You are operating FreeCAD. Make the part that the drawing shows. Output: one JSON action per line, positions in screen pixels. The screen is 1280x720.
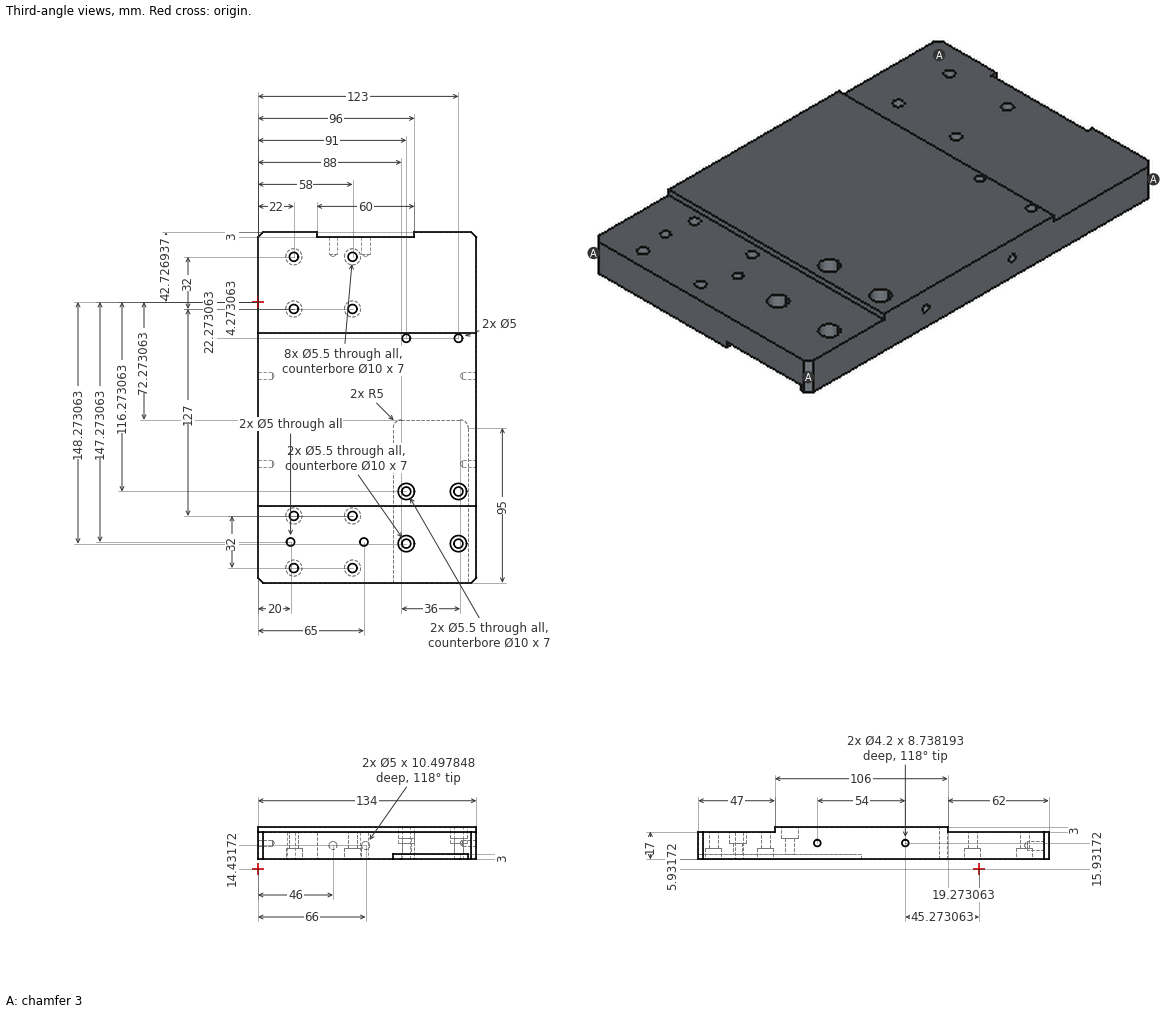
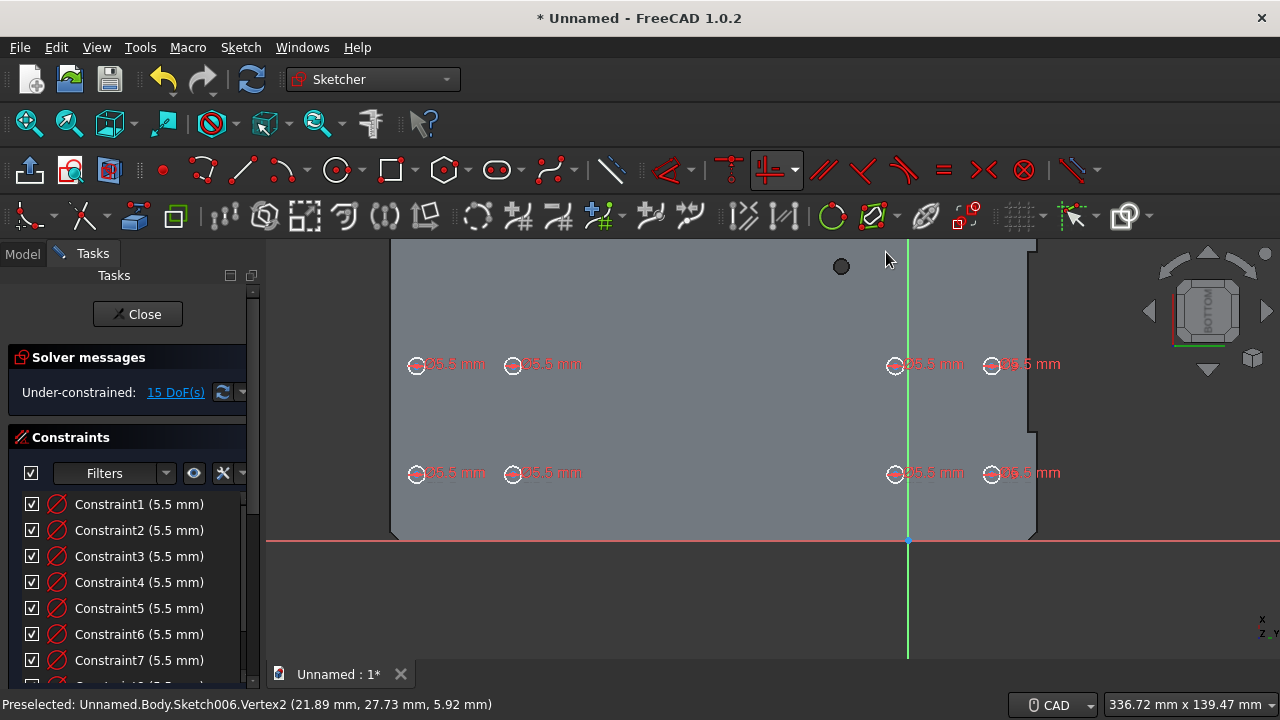
{"action": "left_click", "coordinate": [992, 475]}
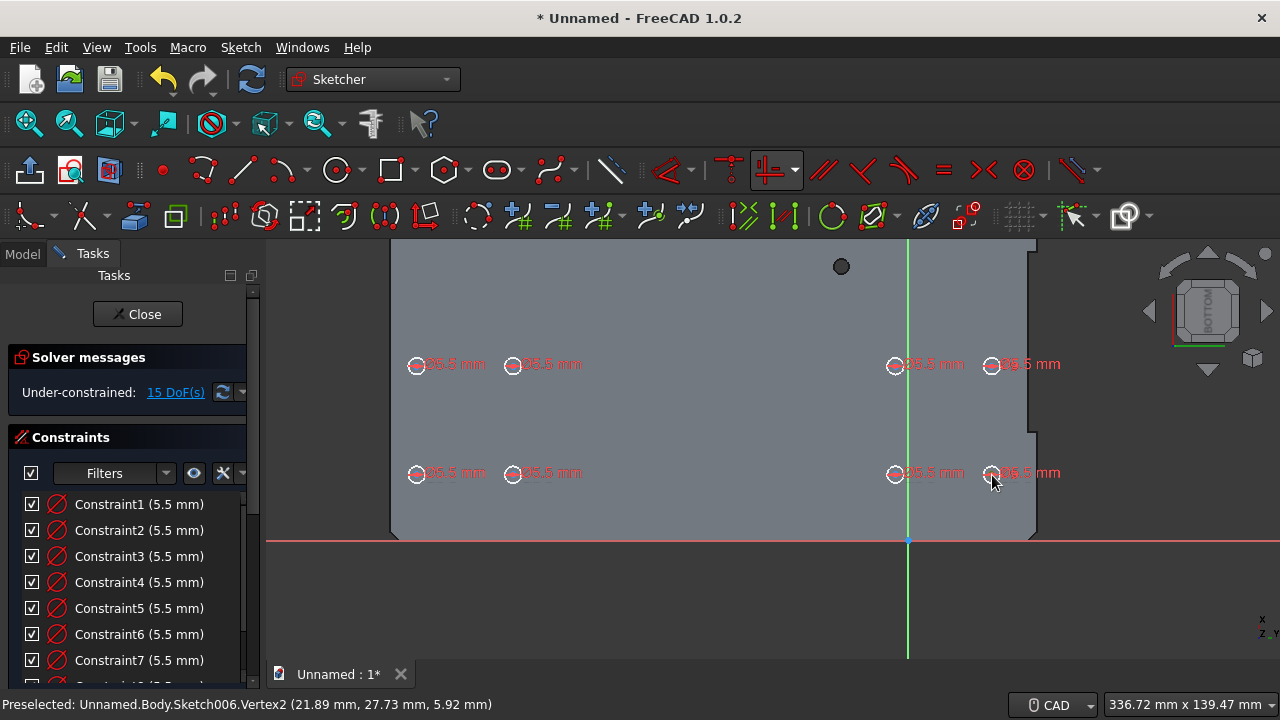
{"action": "left_click", "coordinate": [896, 475]}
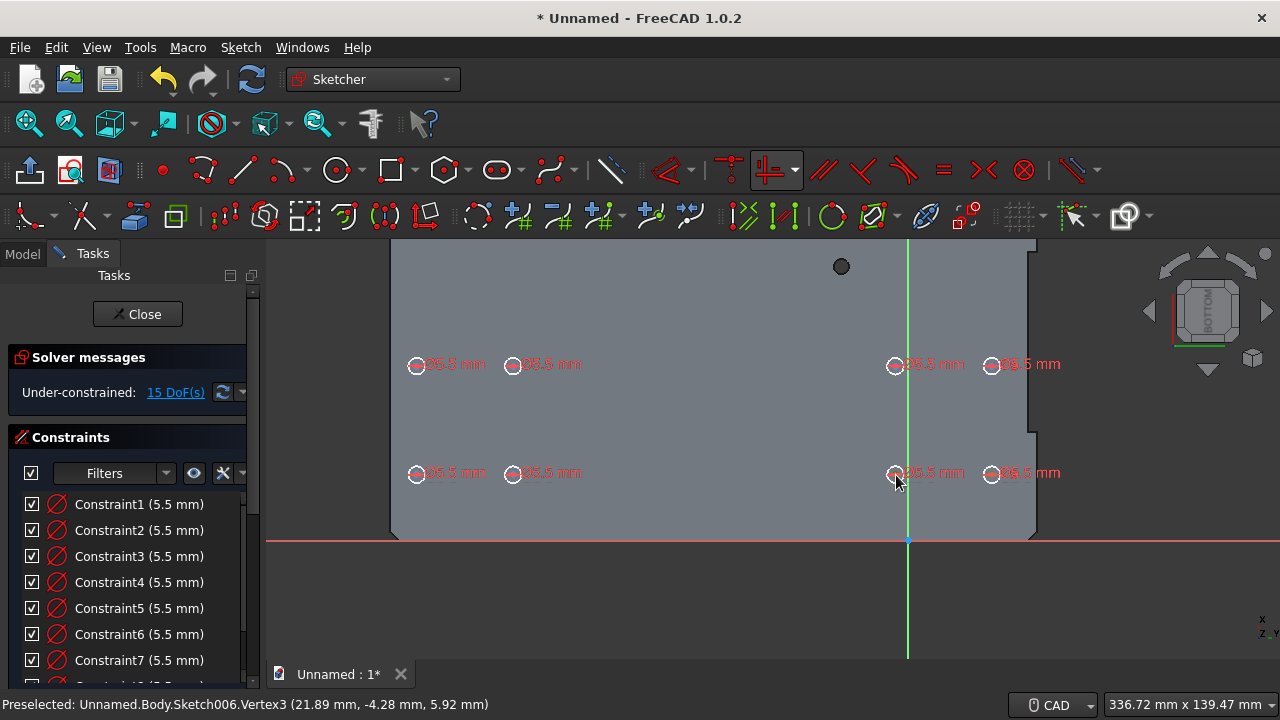
{"action": "left_click", "coordinate": [798, 170]}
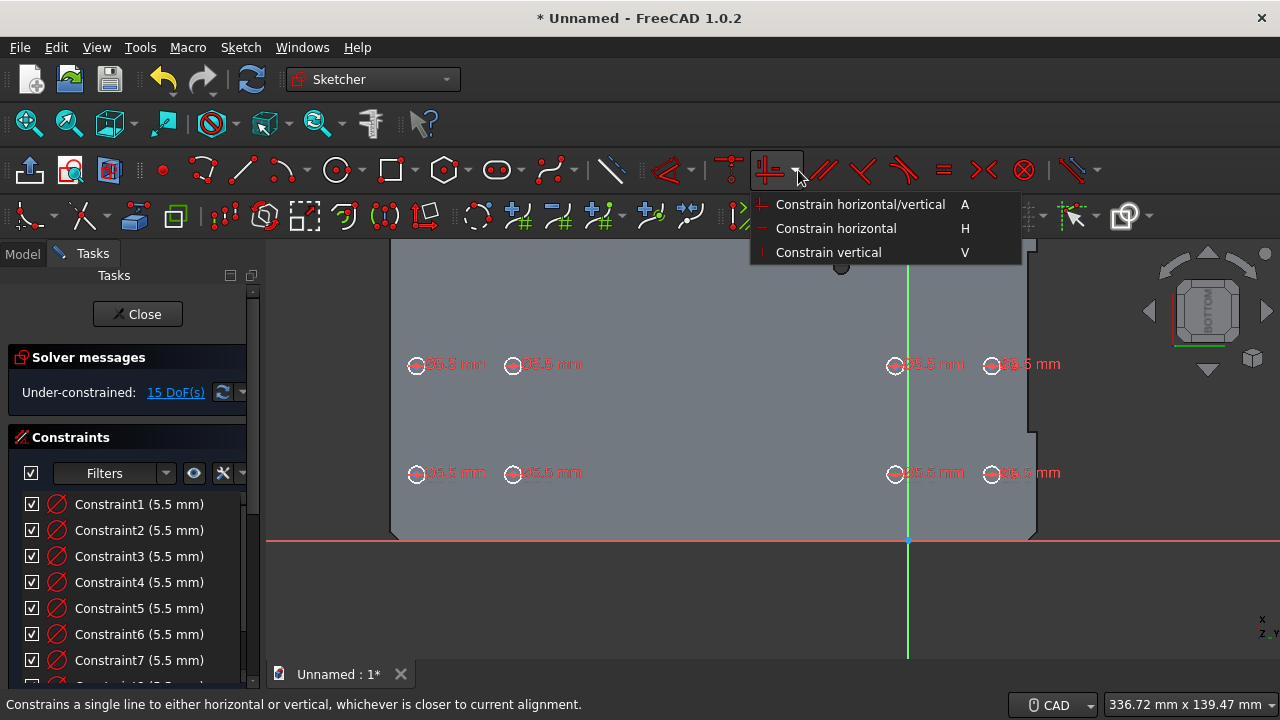
{"action": "left_click", "coordinate": [886, 228]}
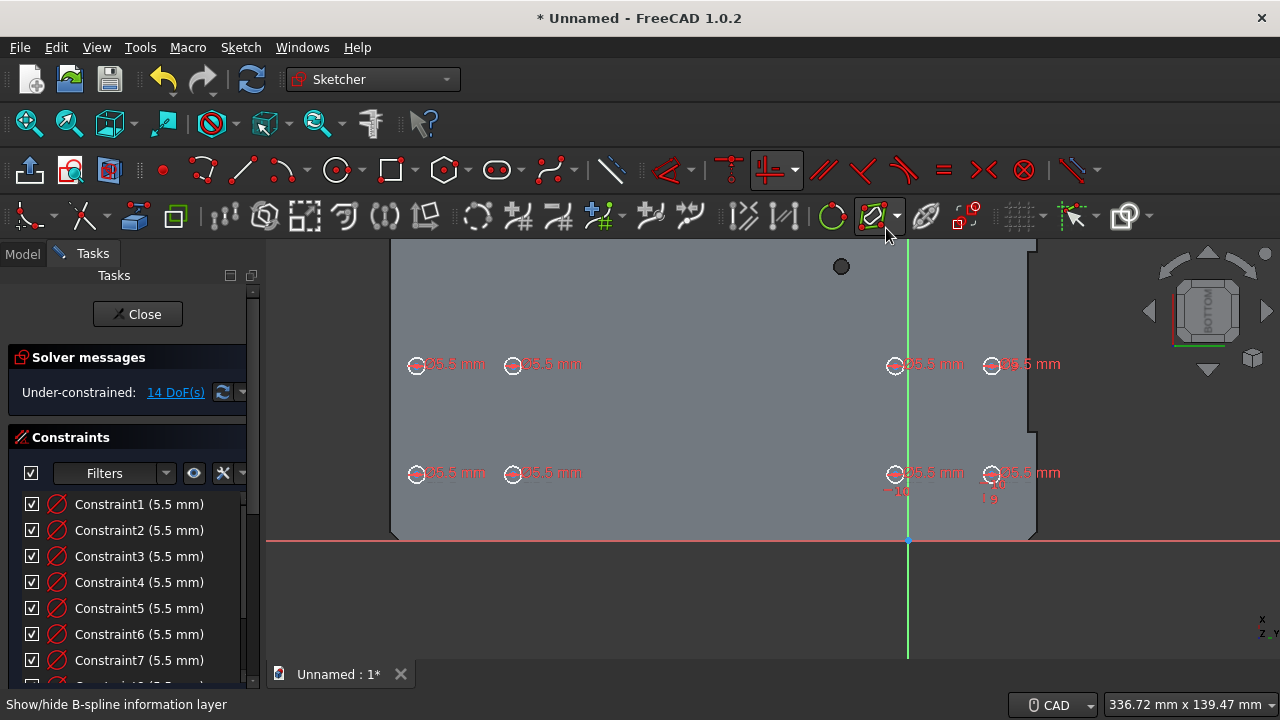
{"action": "left_click", "coordinate": [896, 475]}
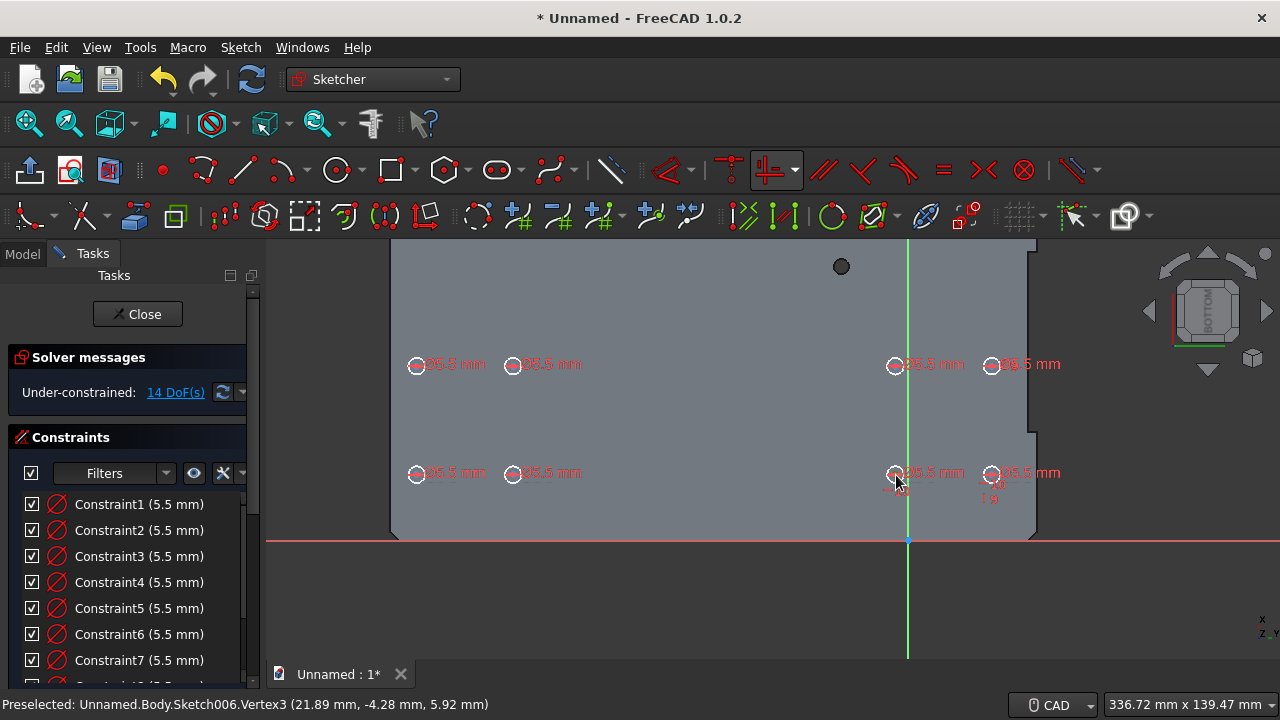
{"action": "left_click", "coordinate": [895, 366]}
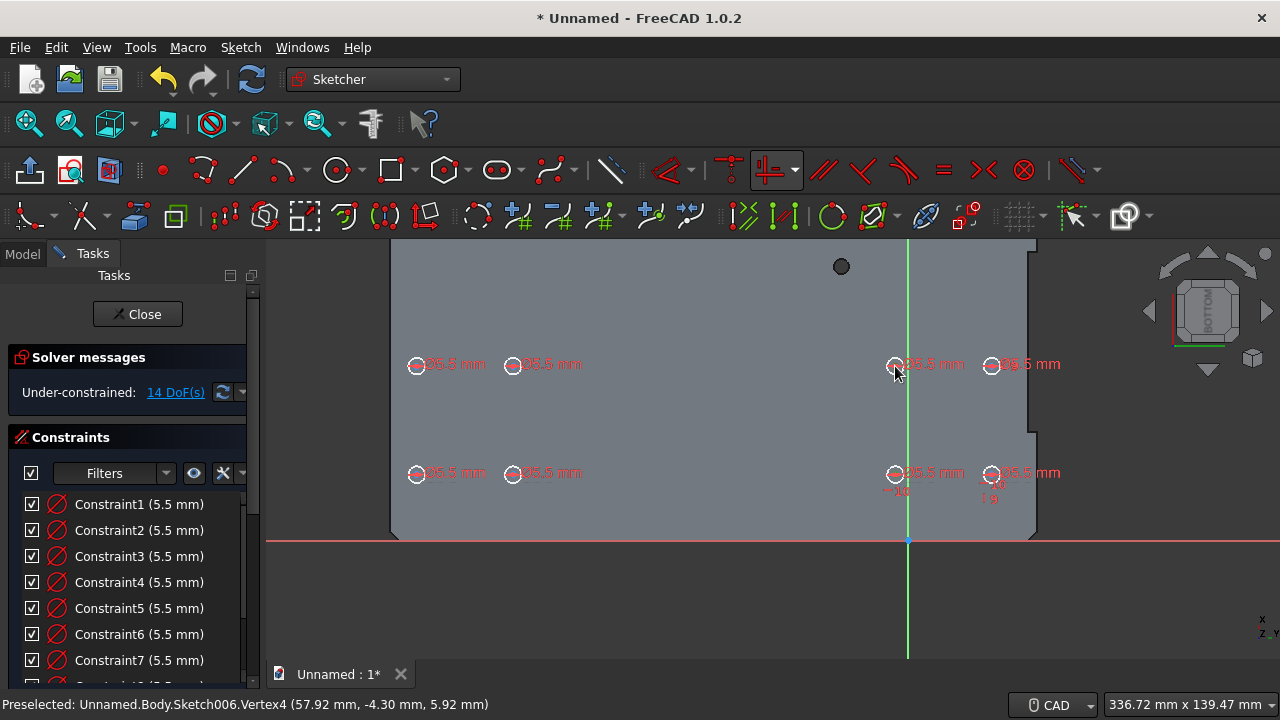
{"action": "left_click", "coordinate": [798, 170]}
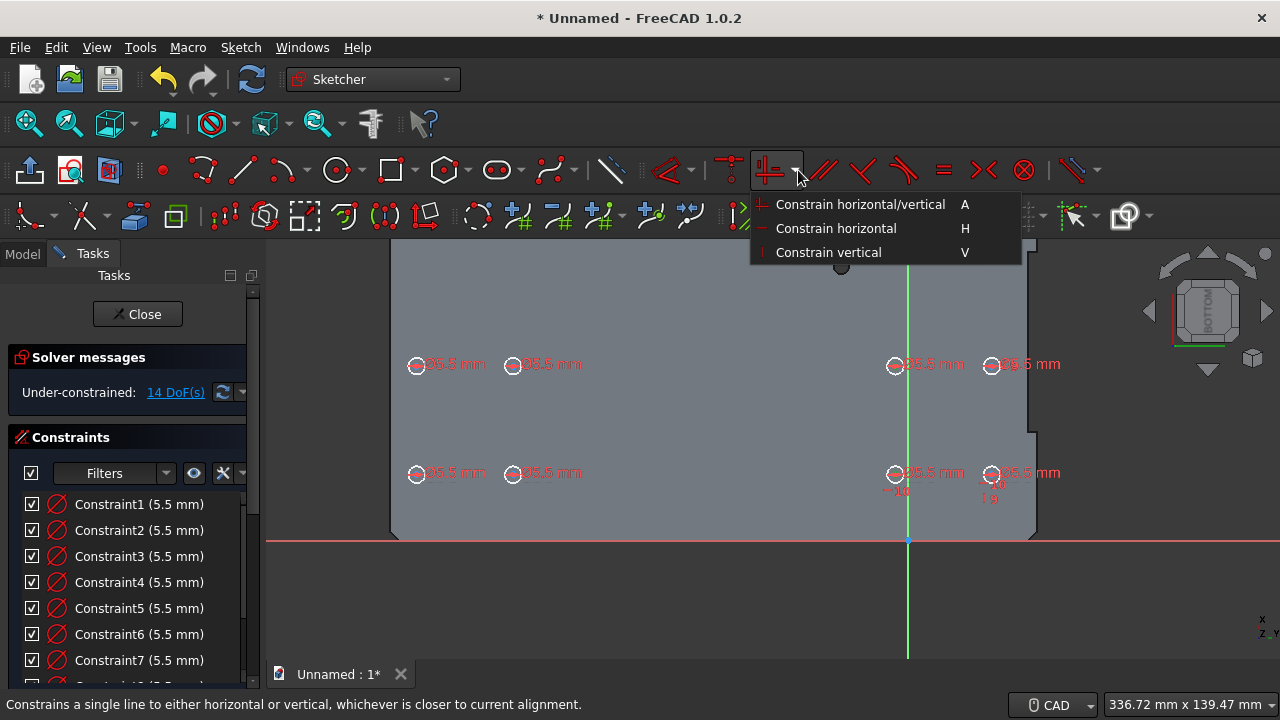
{"action": "left_click", "coordinate": [886, 252]}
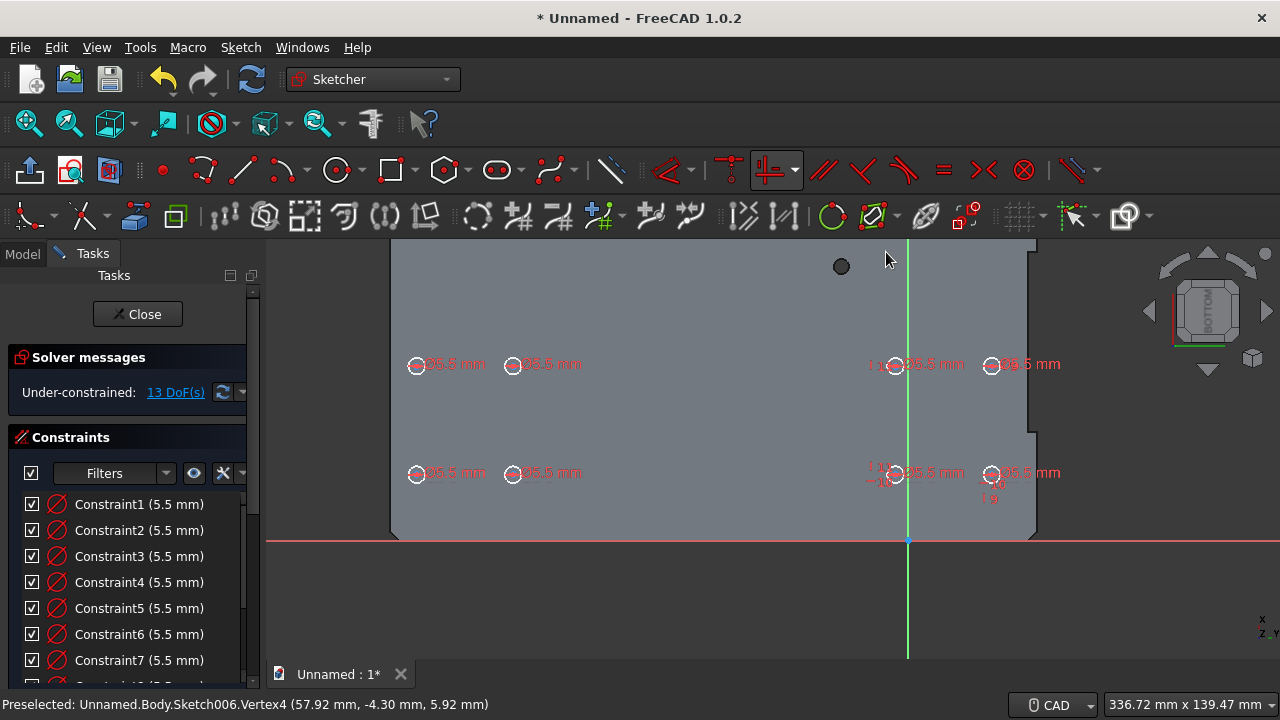
{"action": "left_click", "coordinate": [992, 366]}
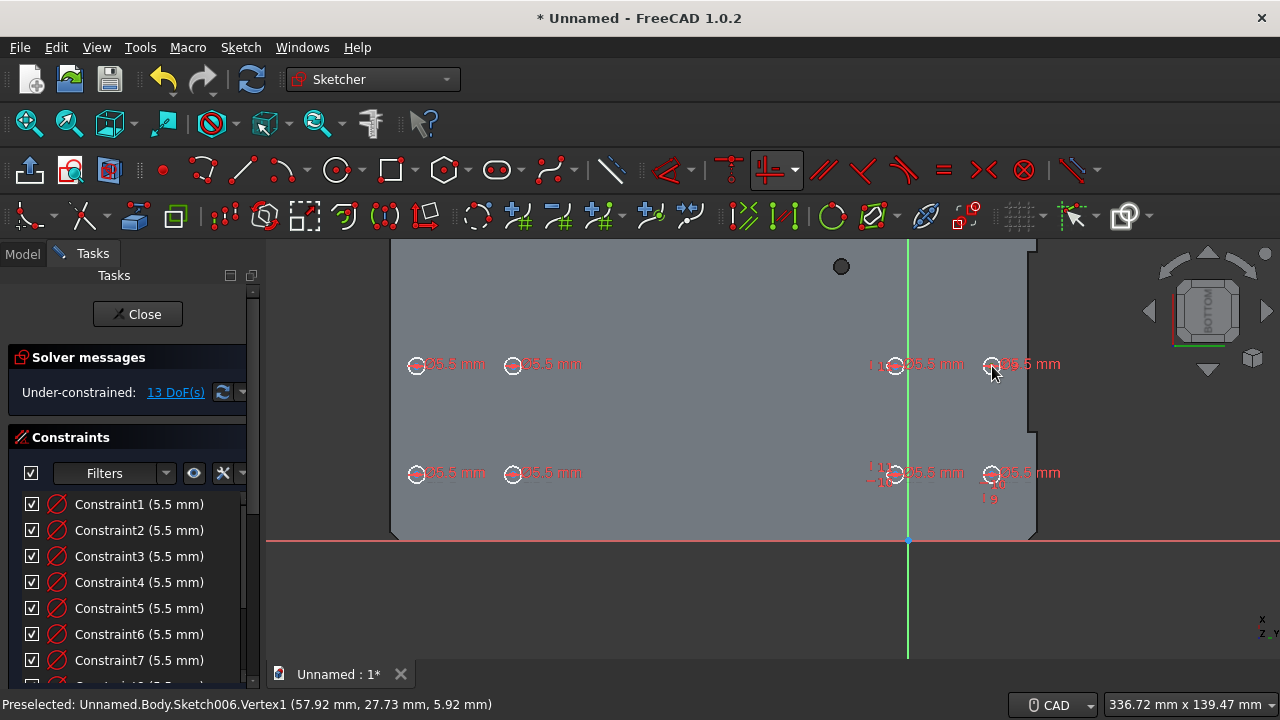
{"action": "left_click", "coordinate": [896, 366]}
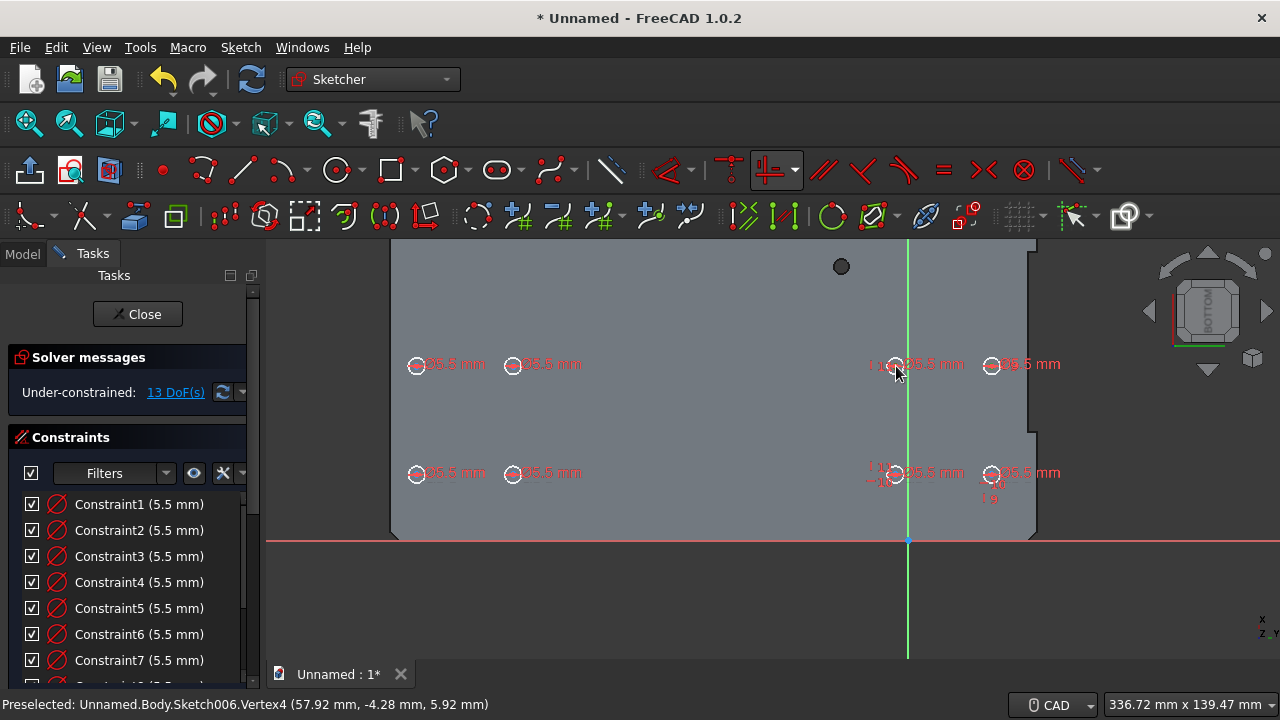
{"action": "key", "text": "h"}